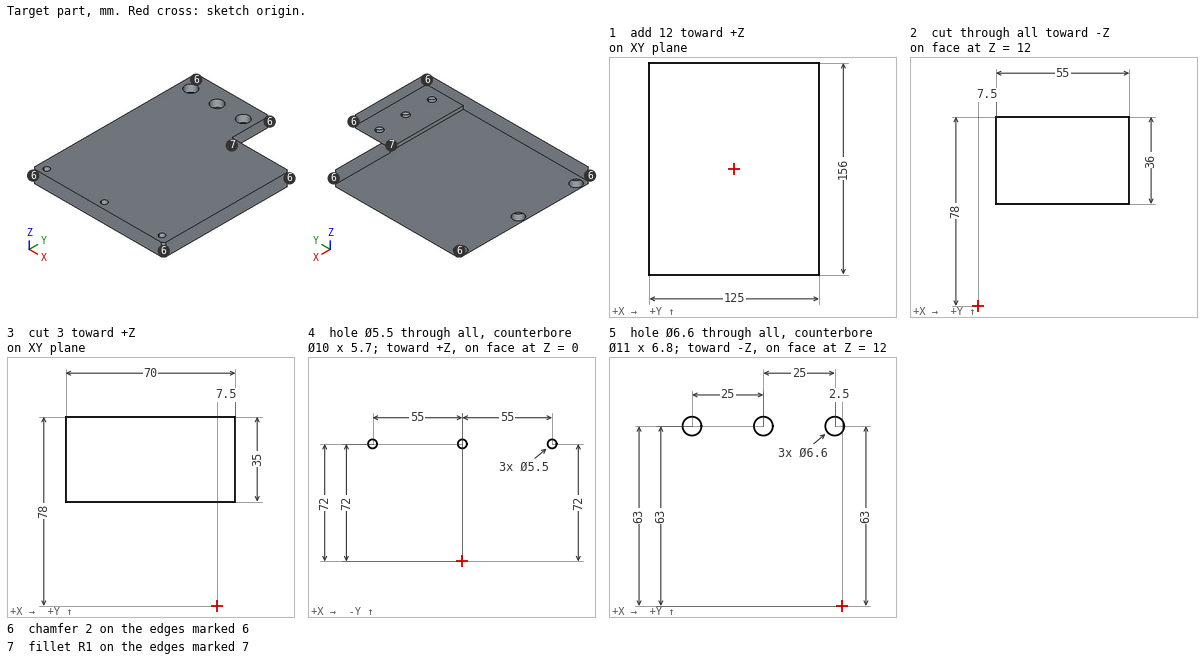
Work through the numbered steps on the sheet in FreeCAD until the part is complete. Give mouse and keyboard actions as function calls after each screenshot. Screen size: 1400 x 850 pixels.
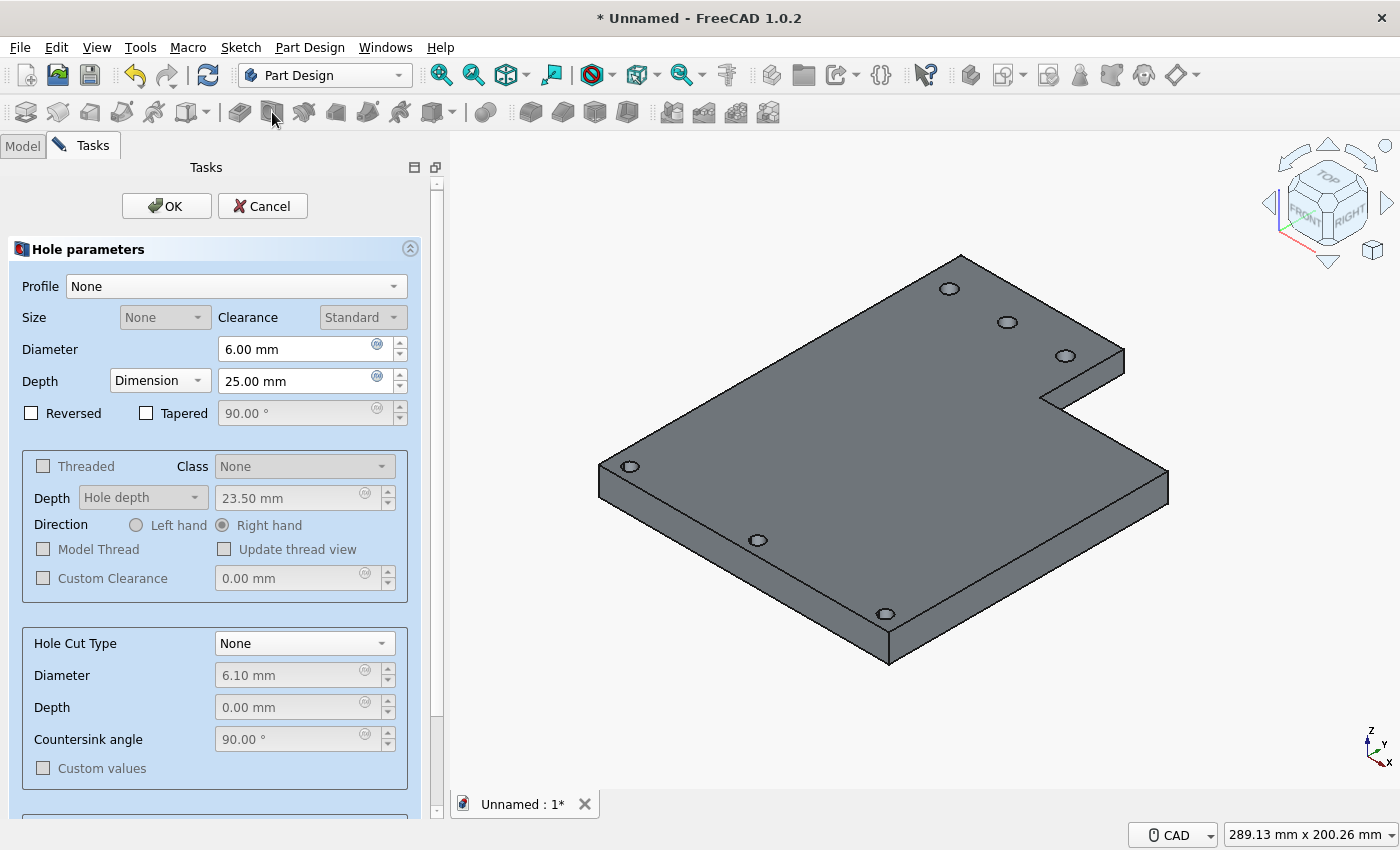
triple_click(305, 349)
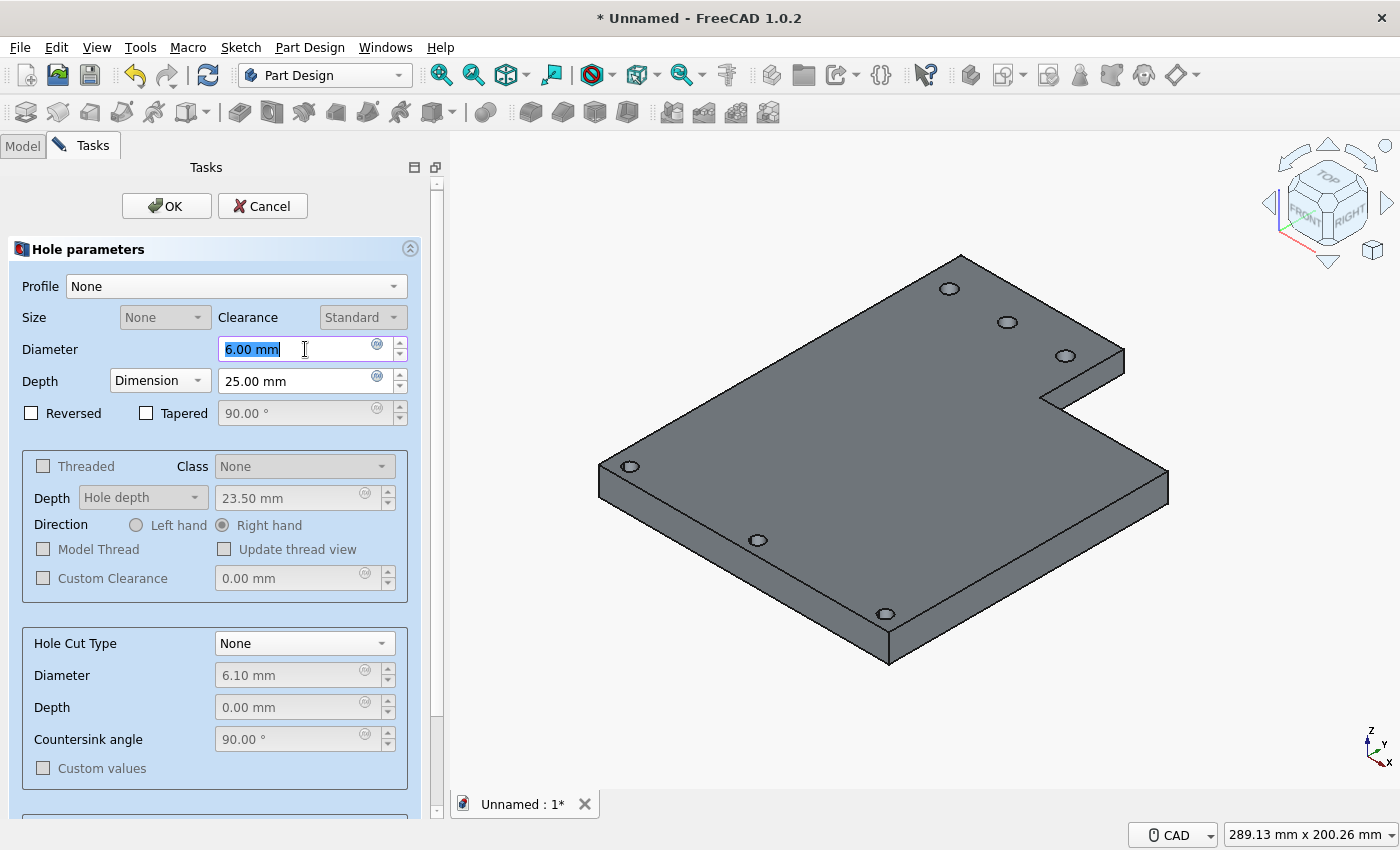
text(6.6)
key(Tab)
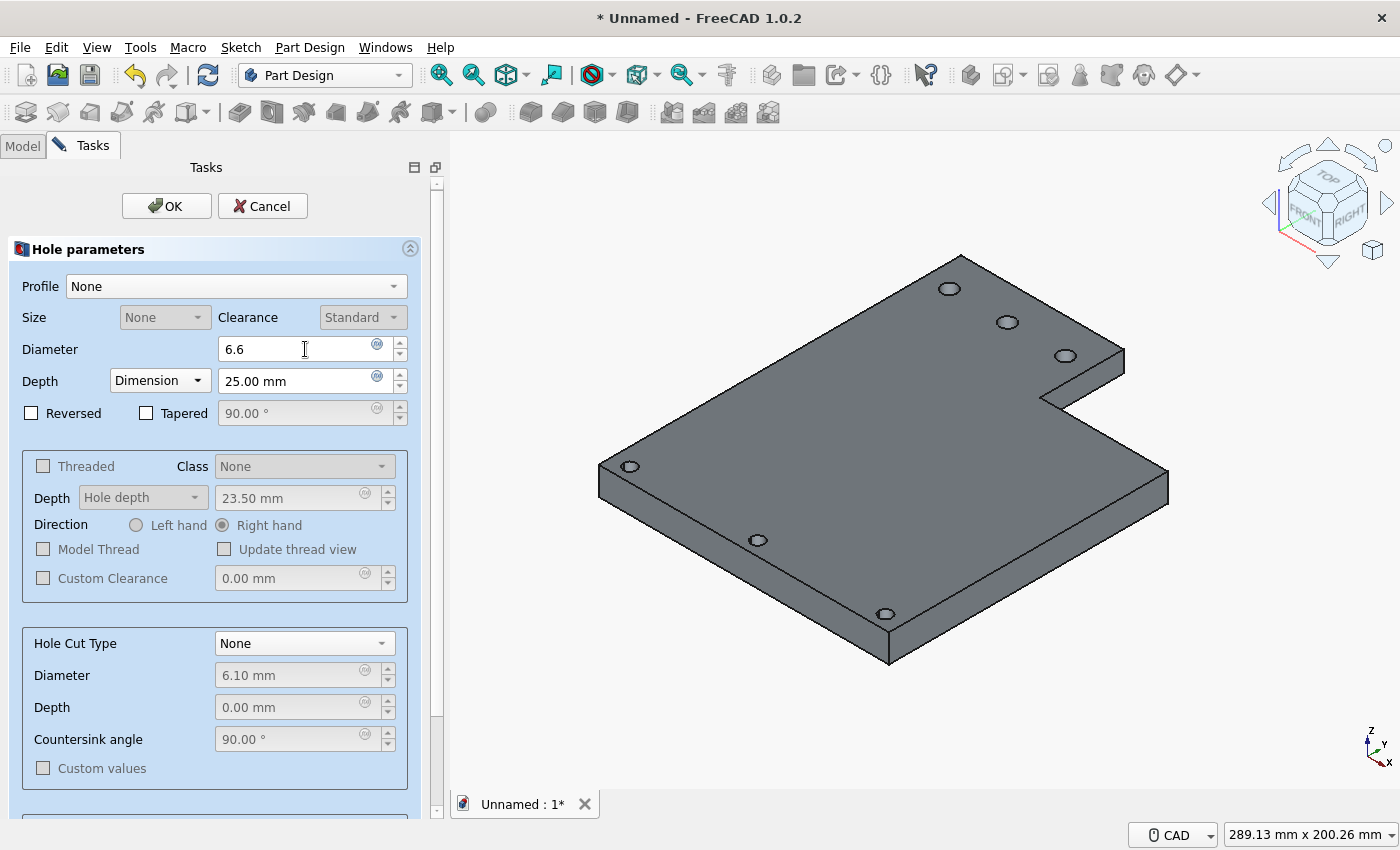
click(161, 380)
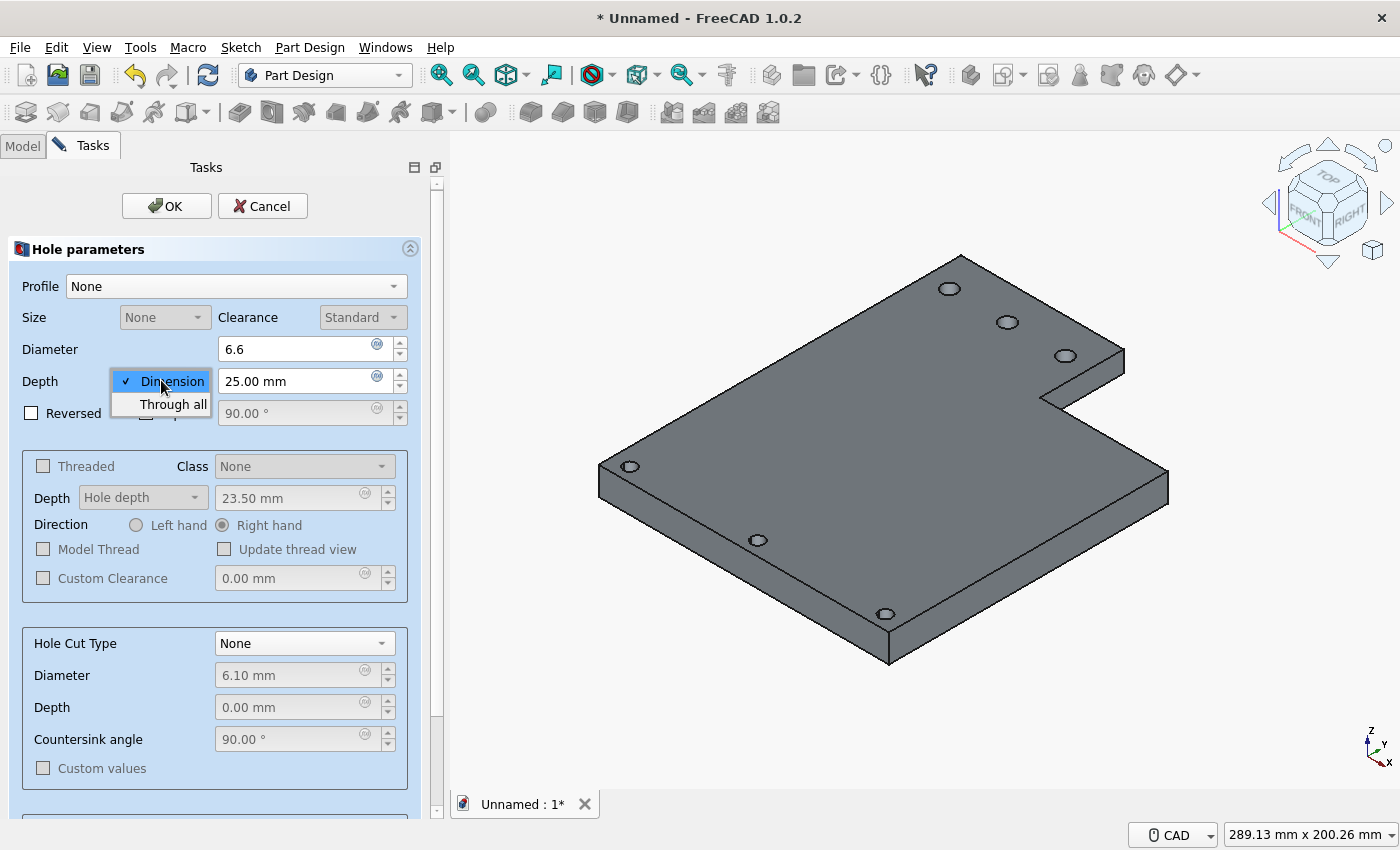
click(160, 404)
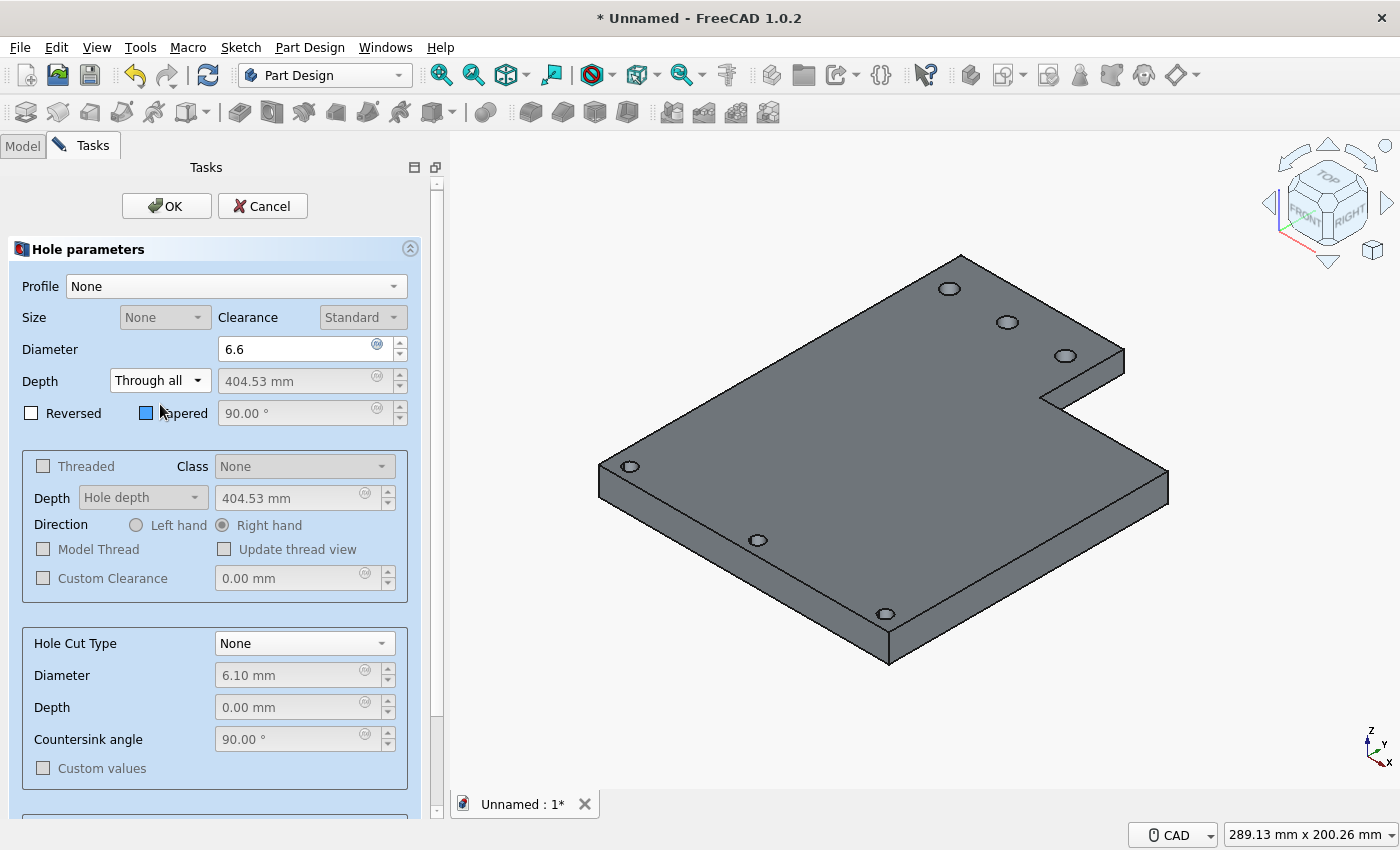
click(306, 644)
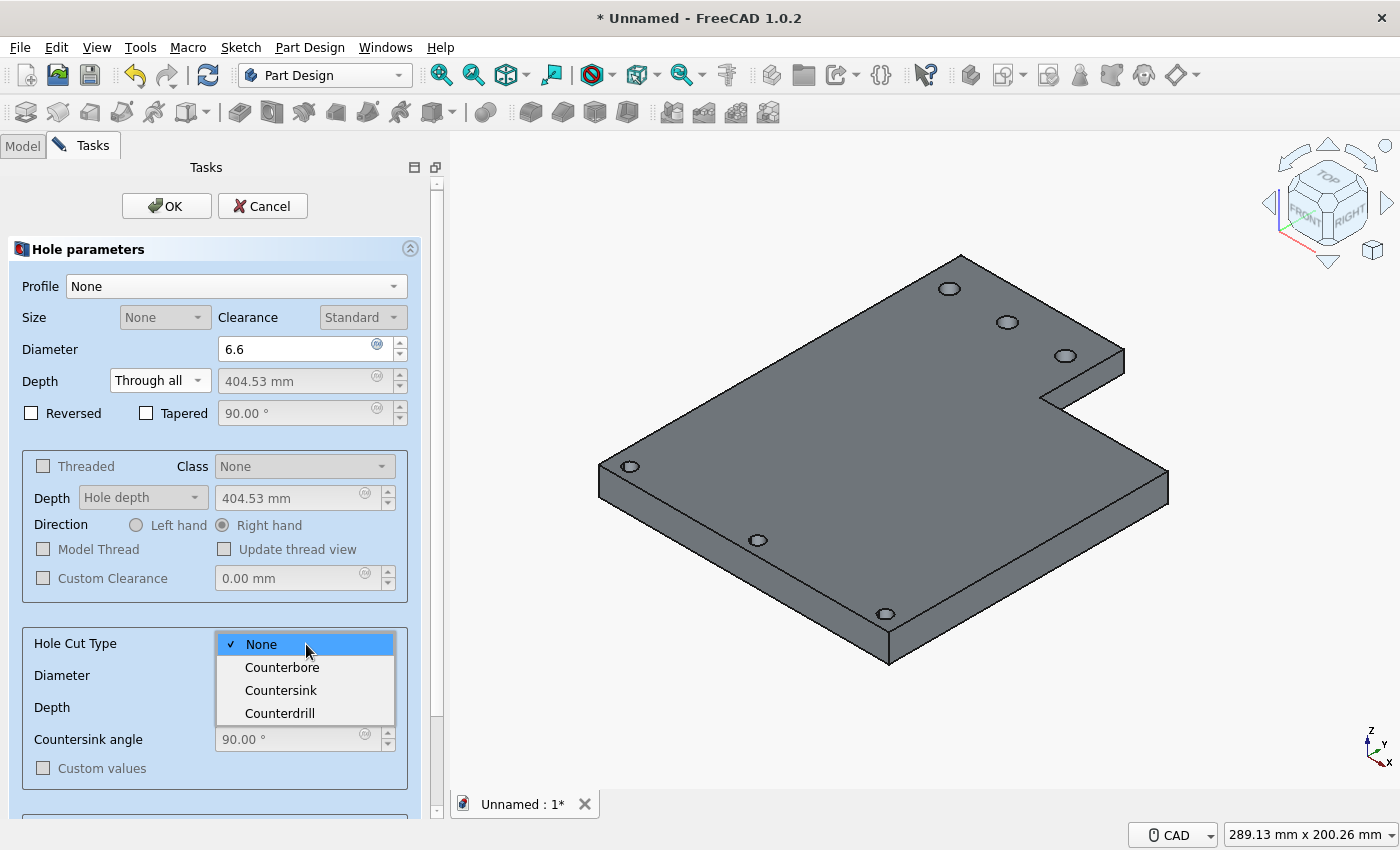
click(304, 668)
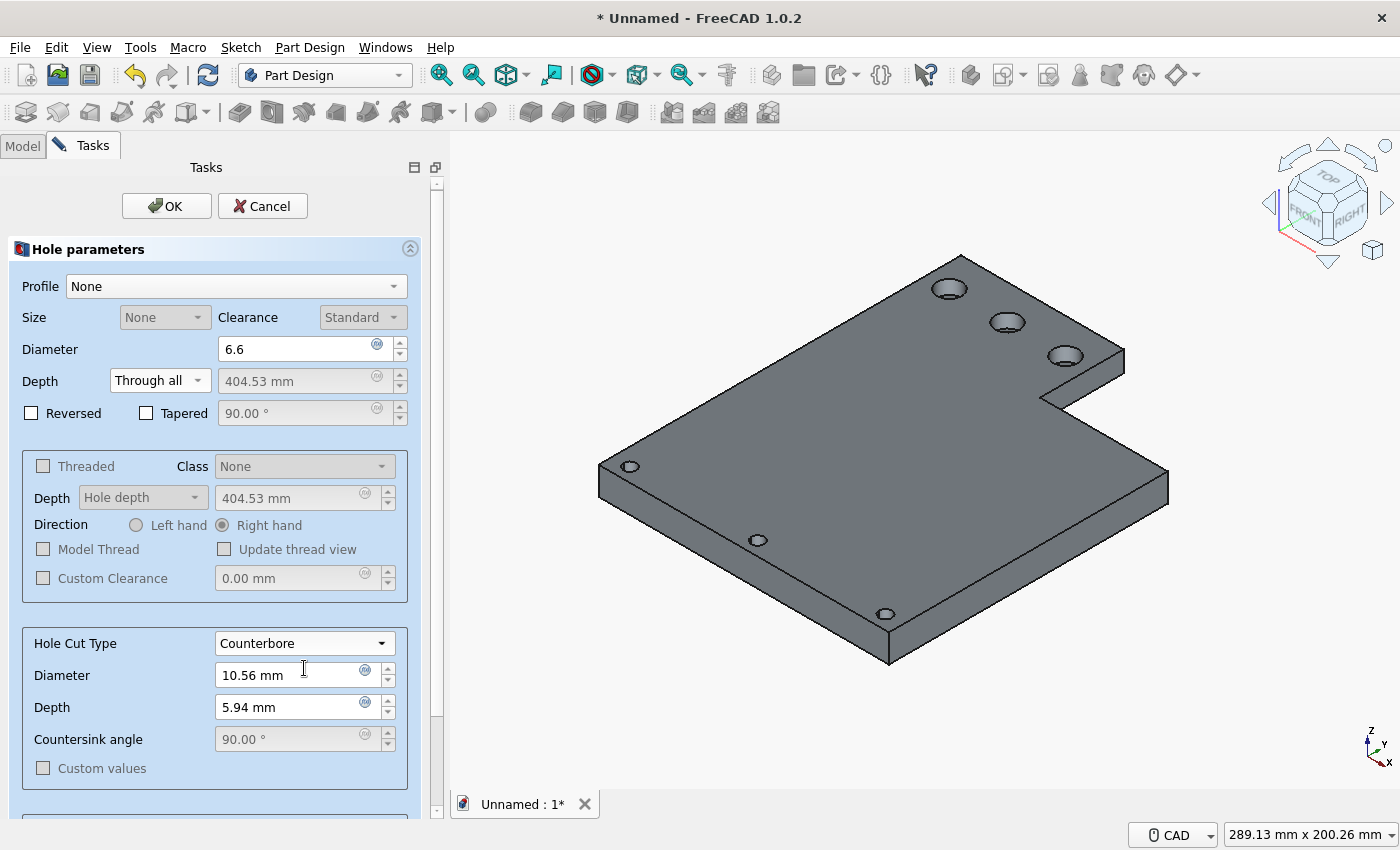
triple_click(298, 675)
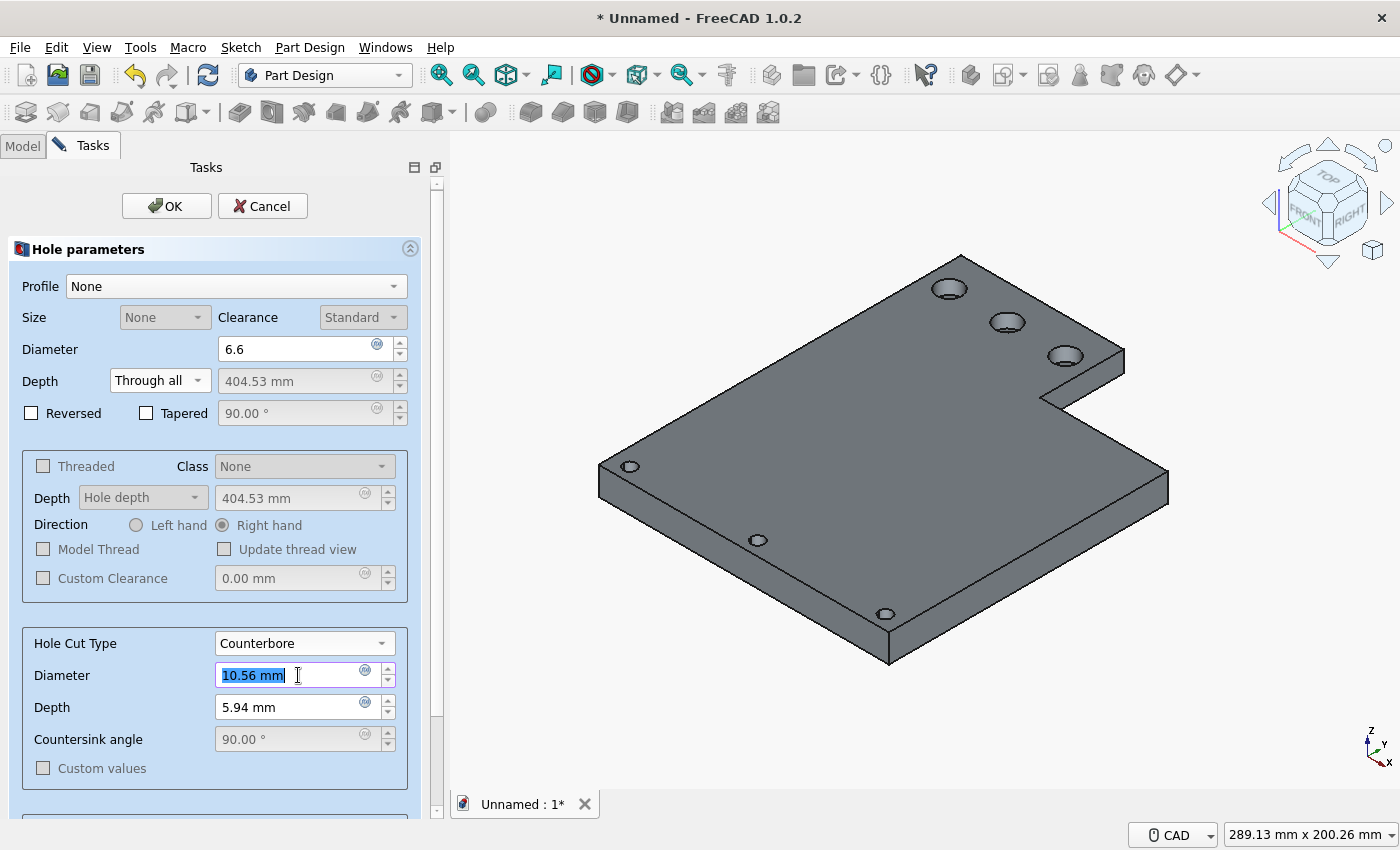
text(11)
key(Tab)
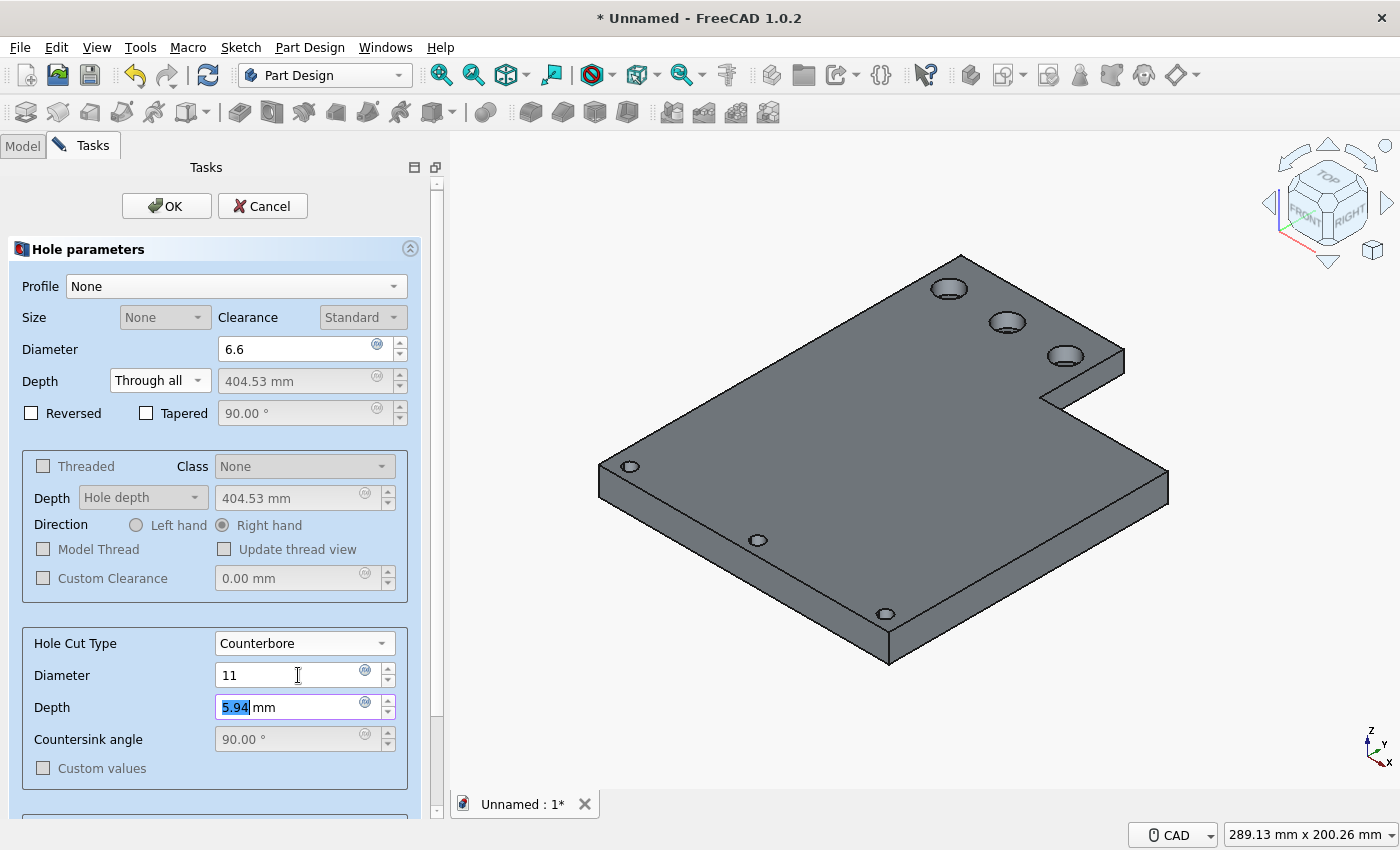
text(6.8)
key(Tab)